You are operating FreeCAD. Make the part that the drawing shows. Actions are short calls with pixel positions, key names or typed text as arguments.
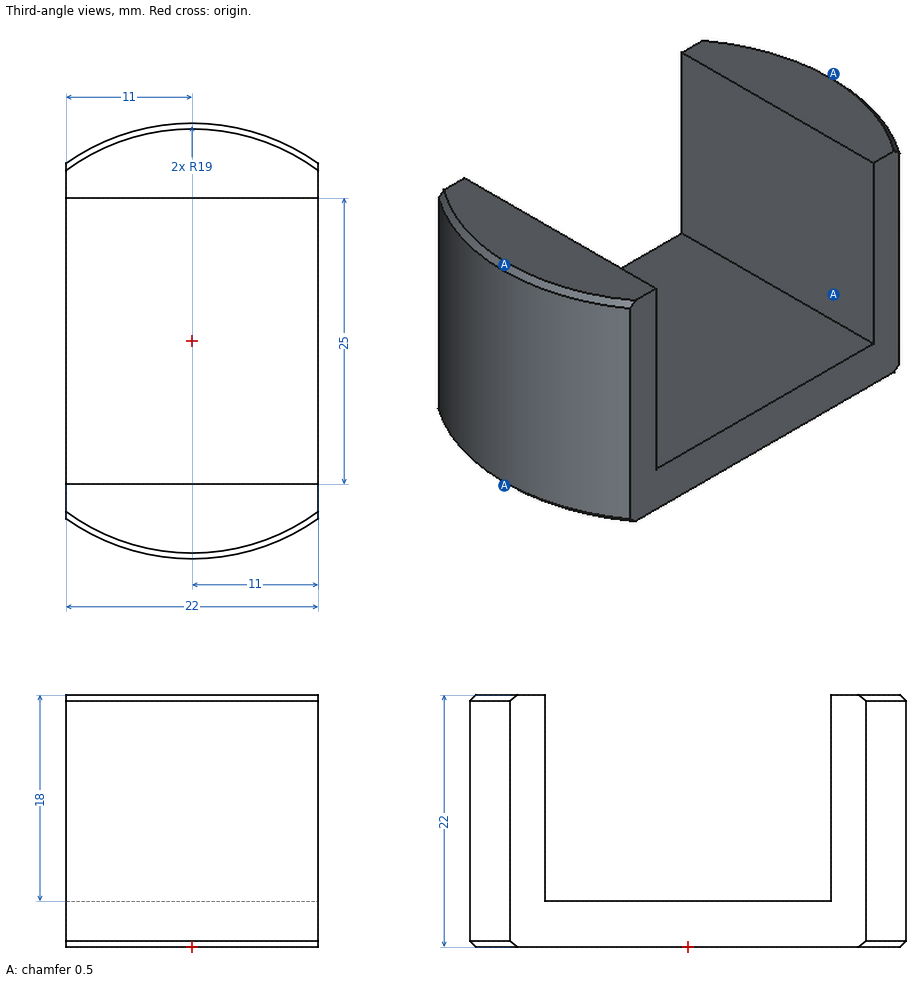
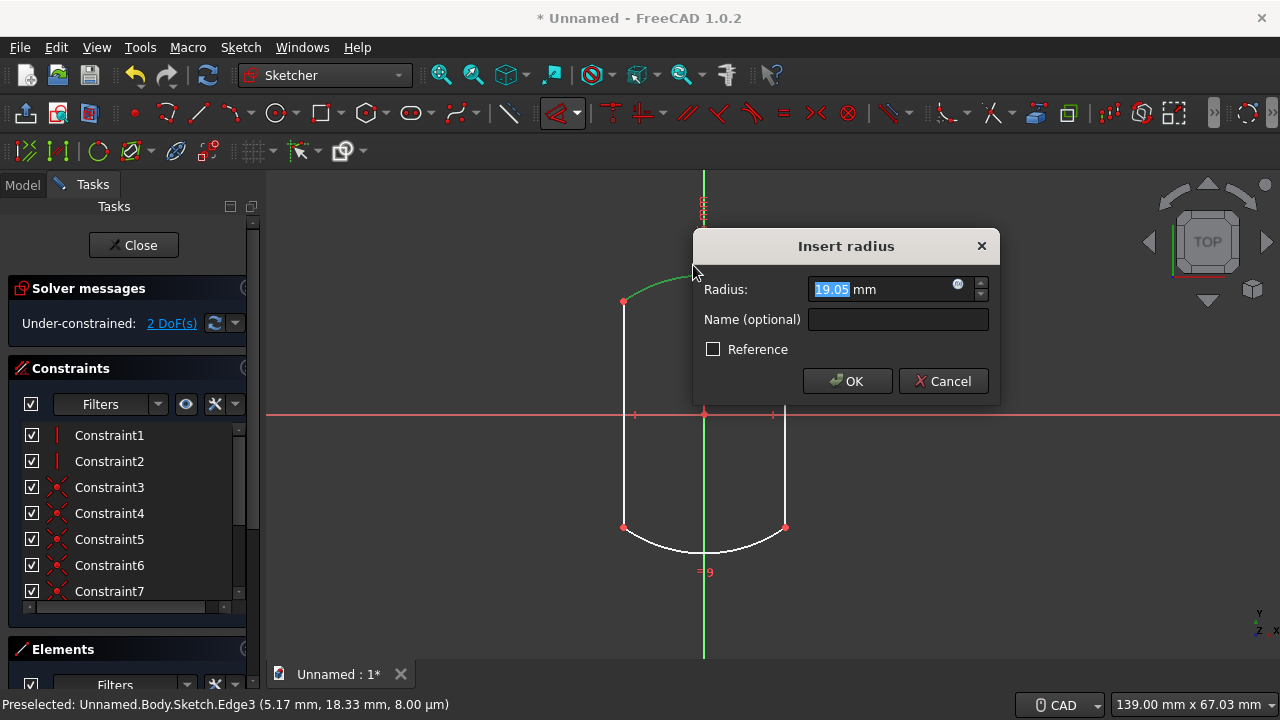
text(19)
key(Return)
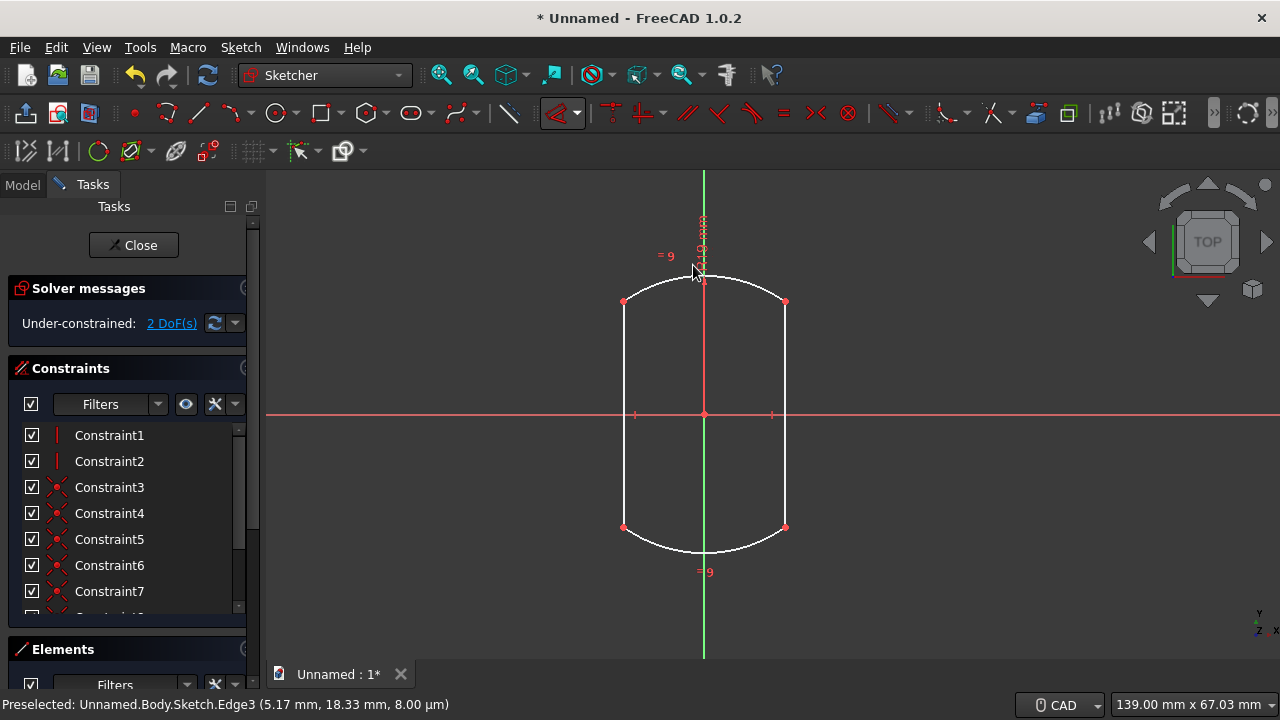
click(785, 527)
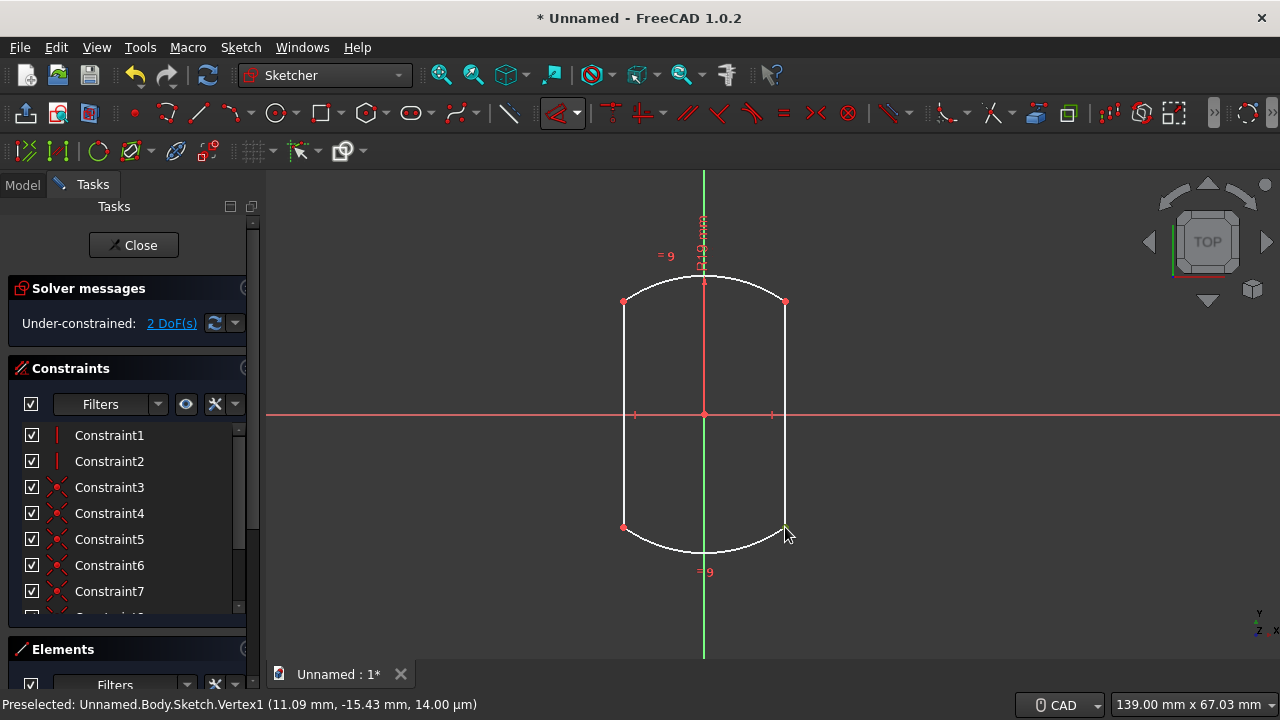
click(580, 114)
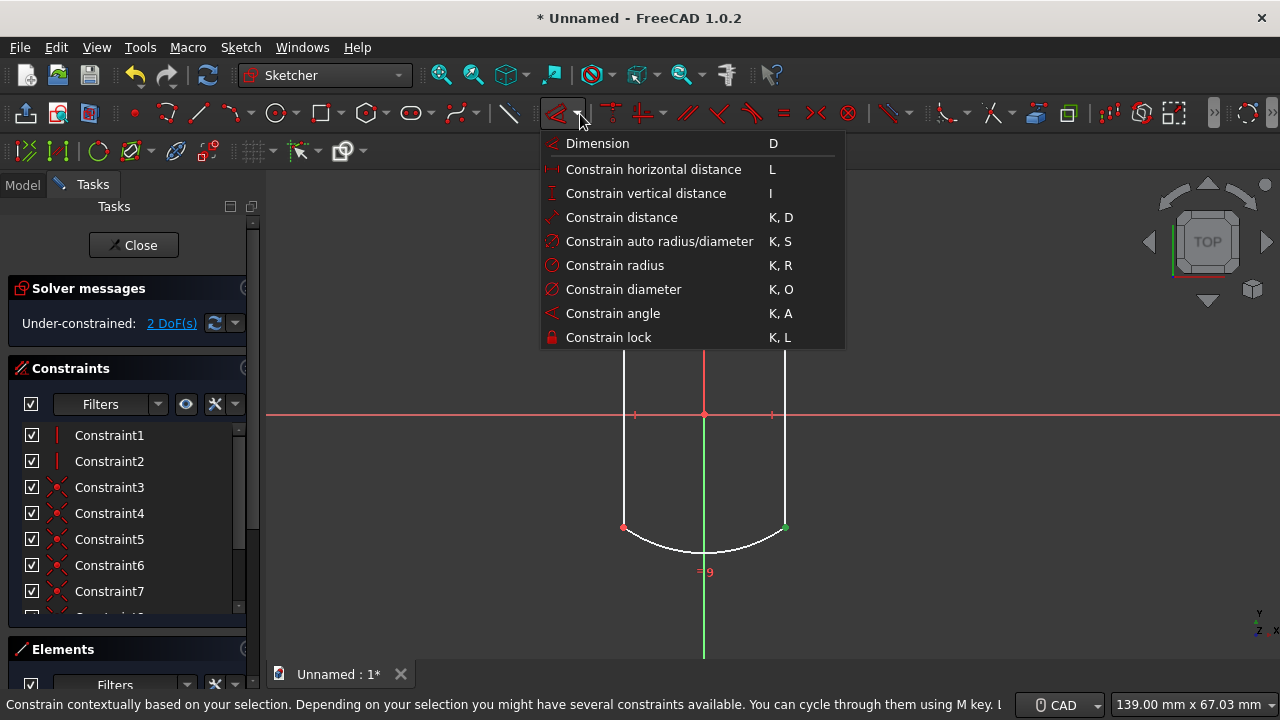
click(693, 169)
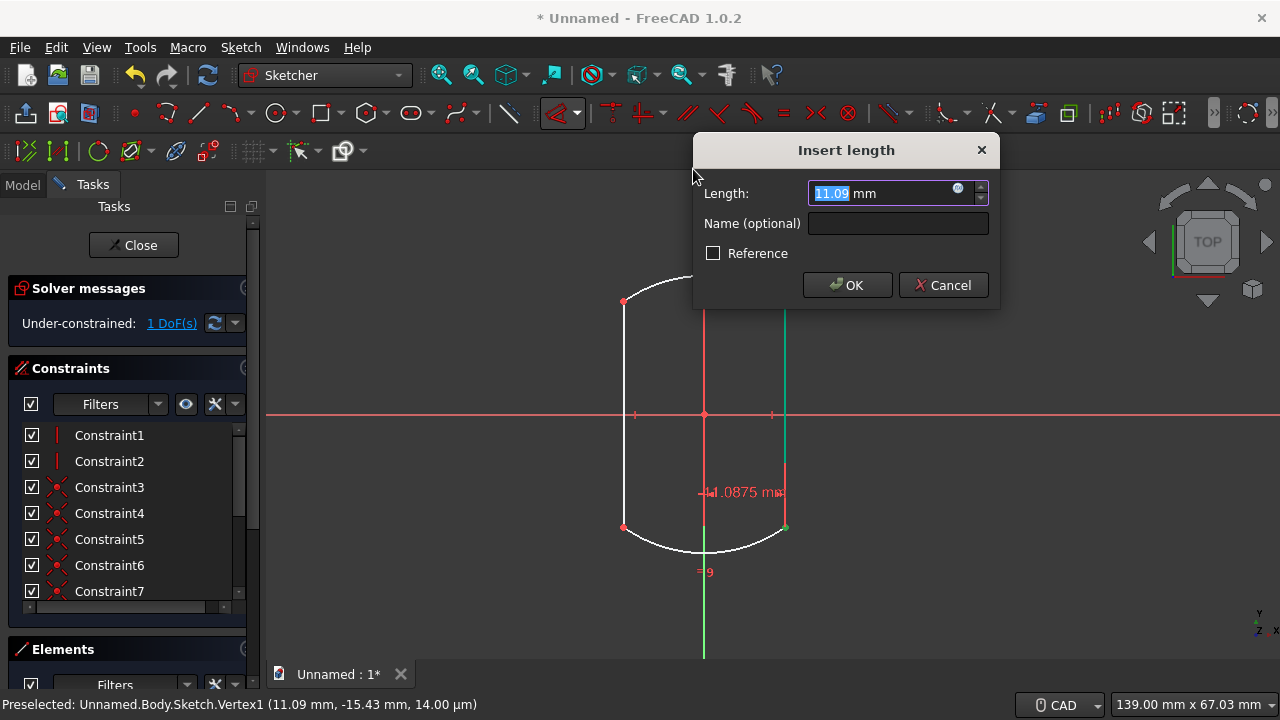
text(11)
key(Return)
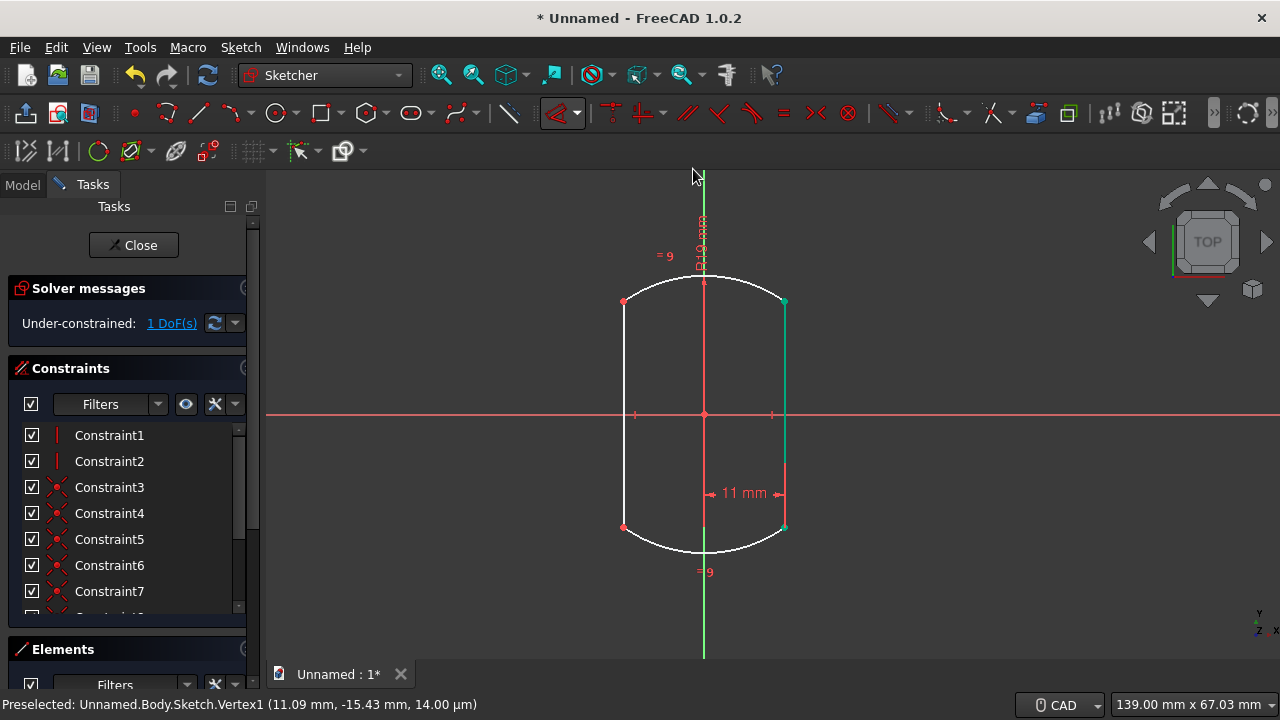
click(624, 302)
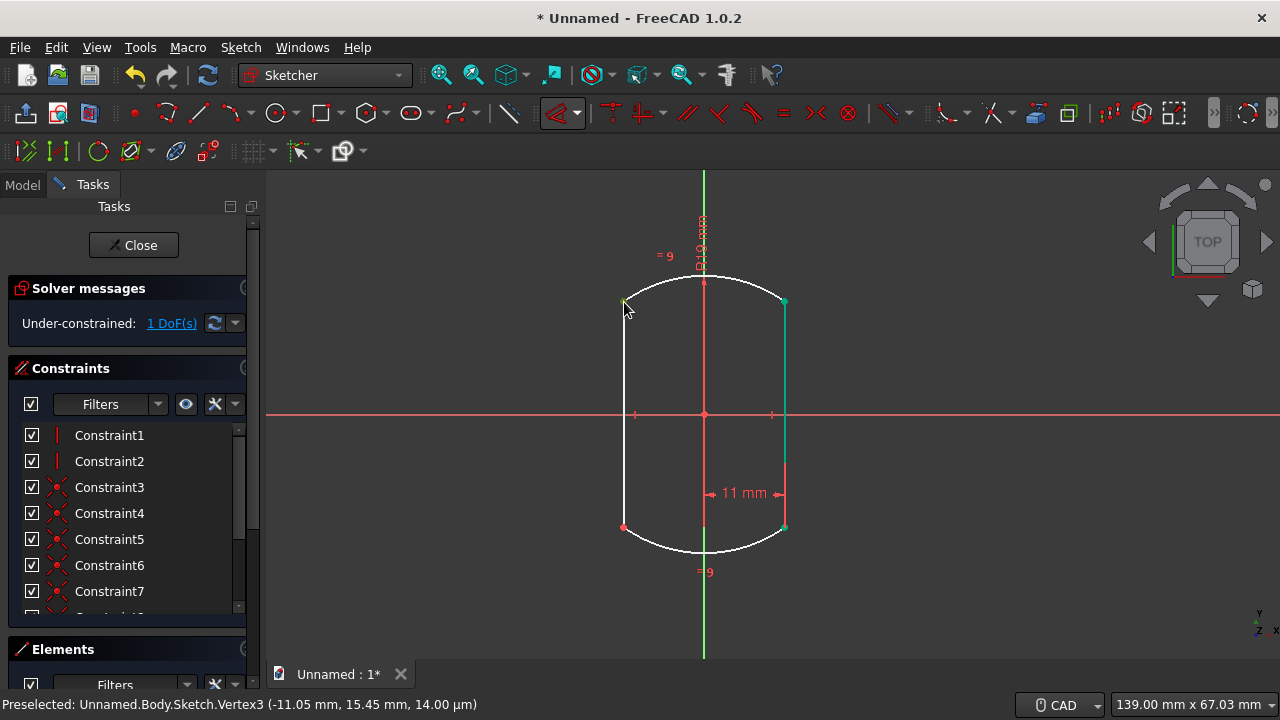
click(580, 114)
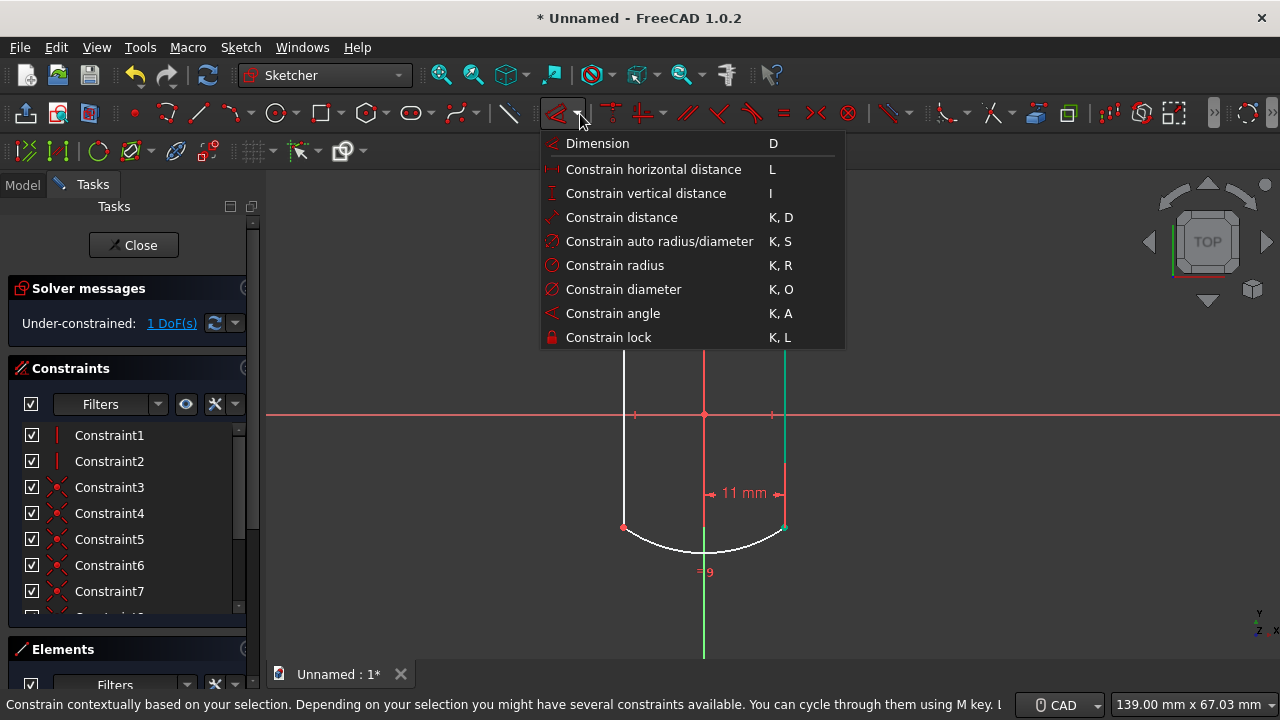
click(693, 169)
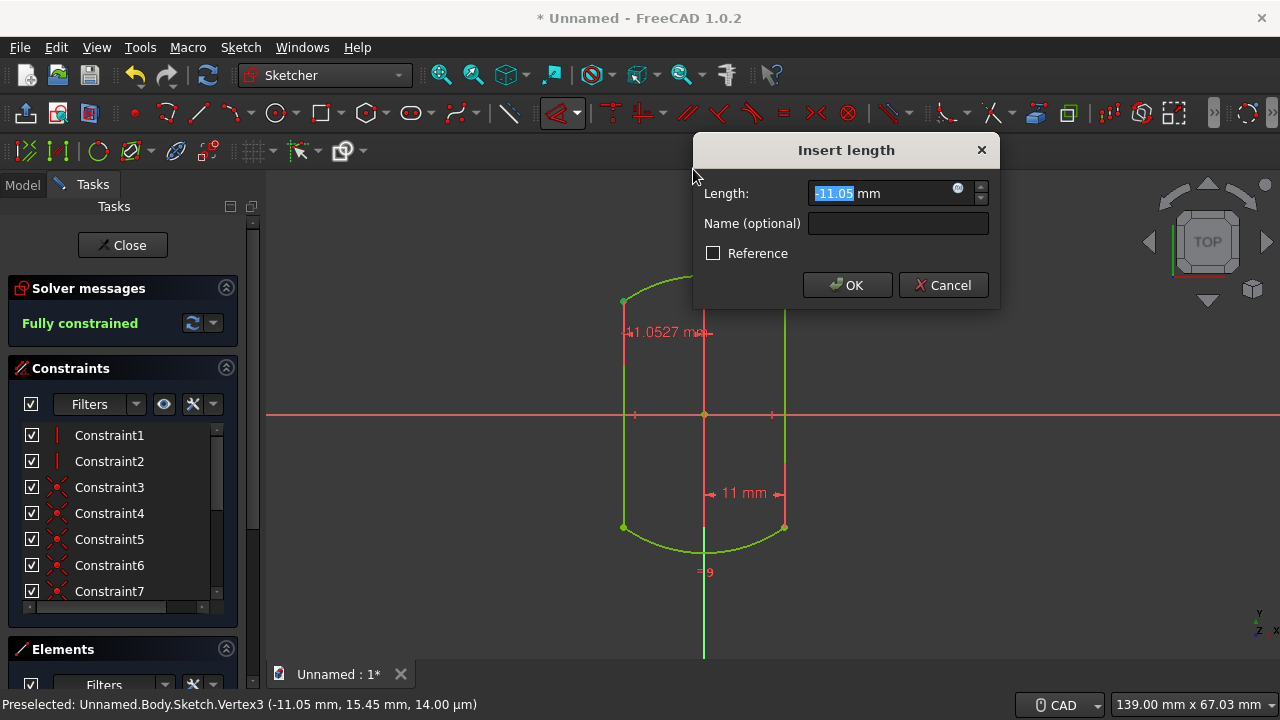
text(-11)
key(Return)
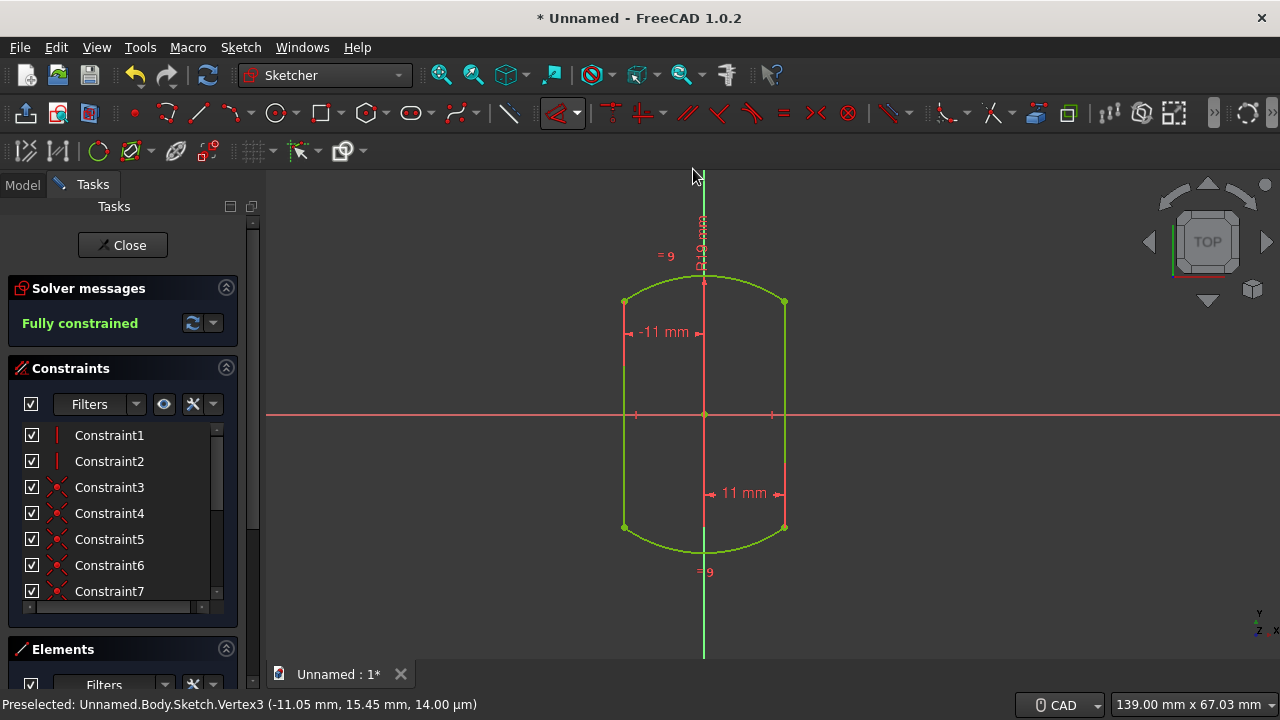
click(123, 245)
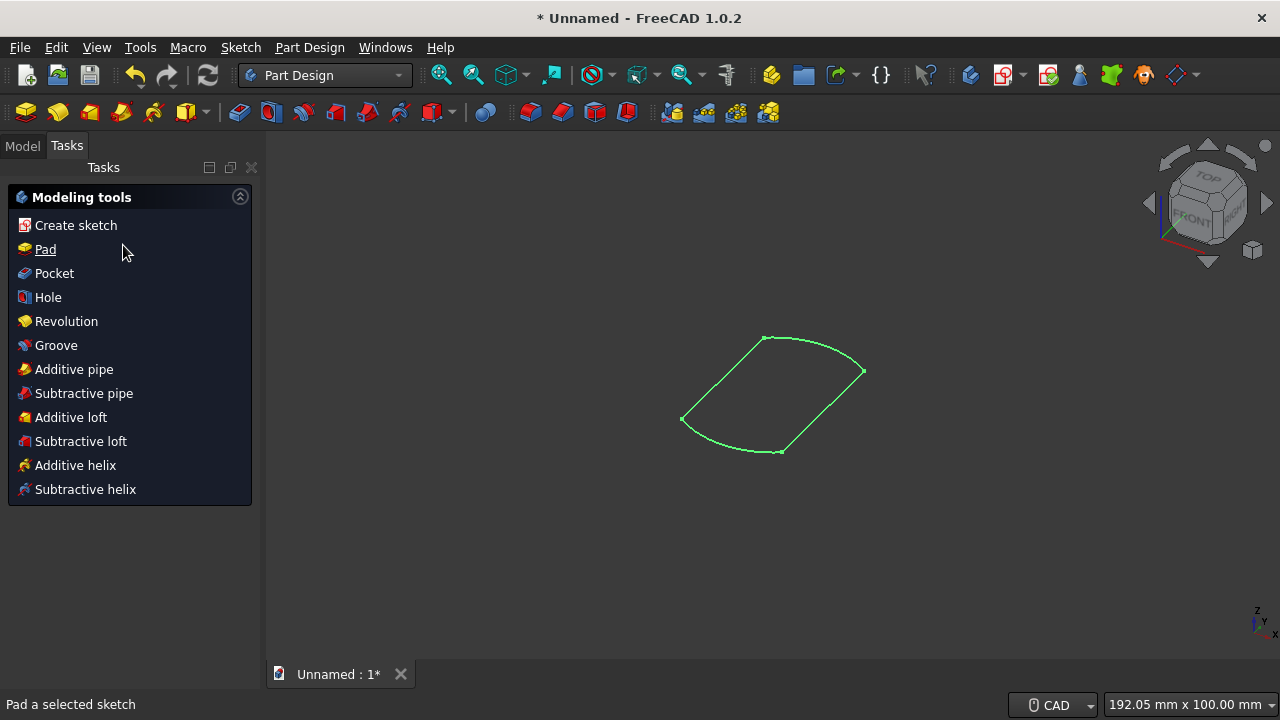
click(26, 112)